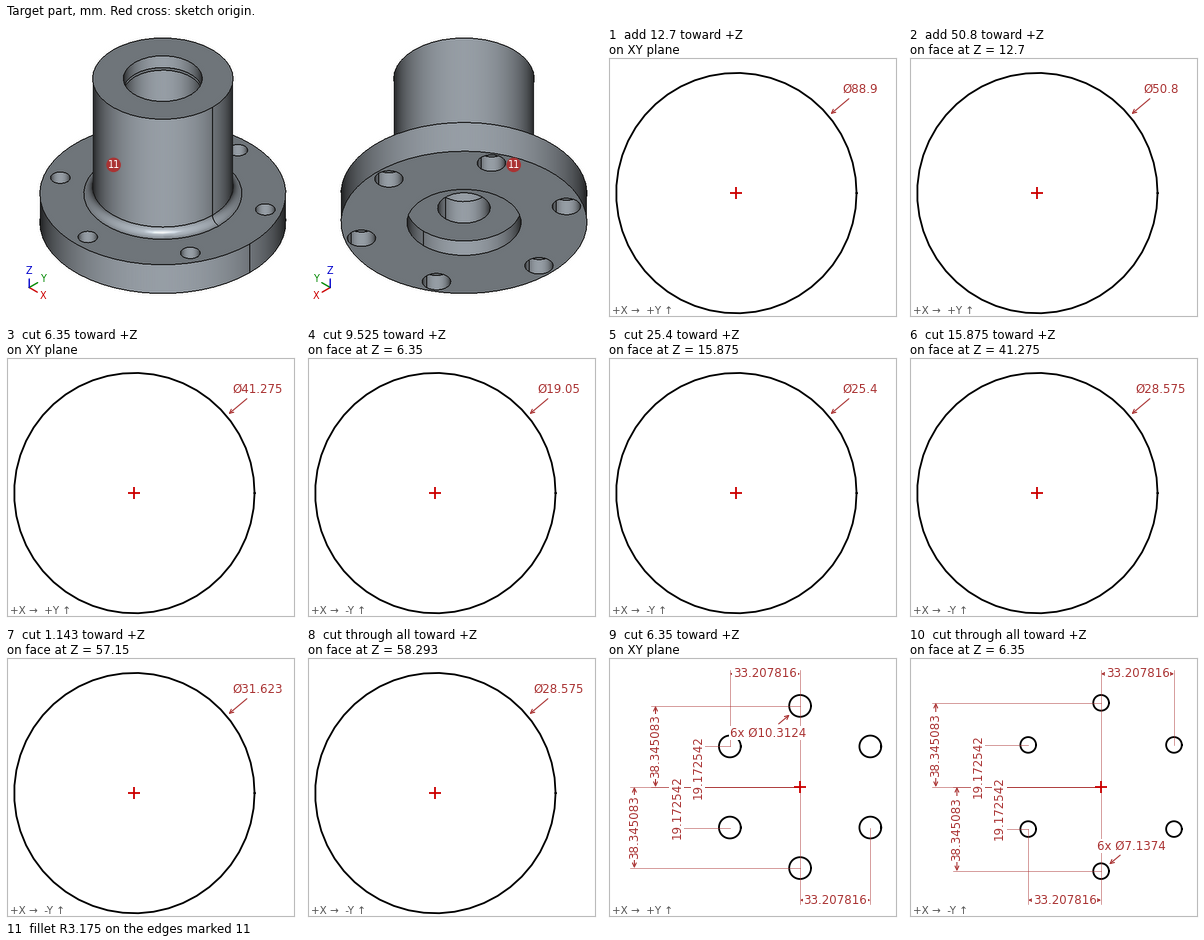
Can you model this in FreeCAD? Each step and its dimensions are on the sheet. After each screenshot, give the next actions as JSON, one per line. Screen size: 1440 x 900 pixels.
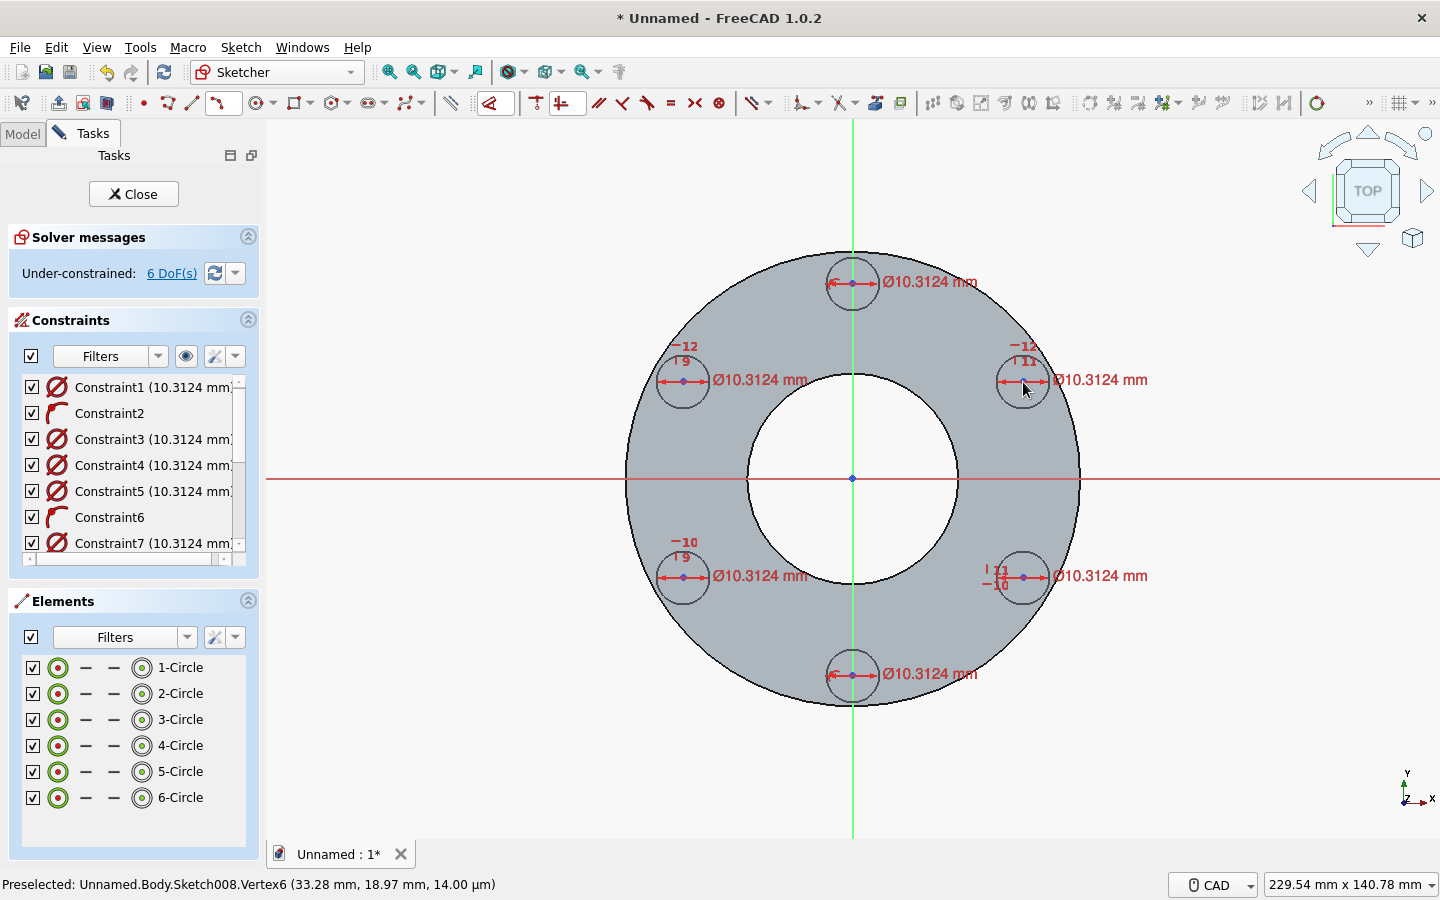
{"action": "key", "text": "d"}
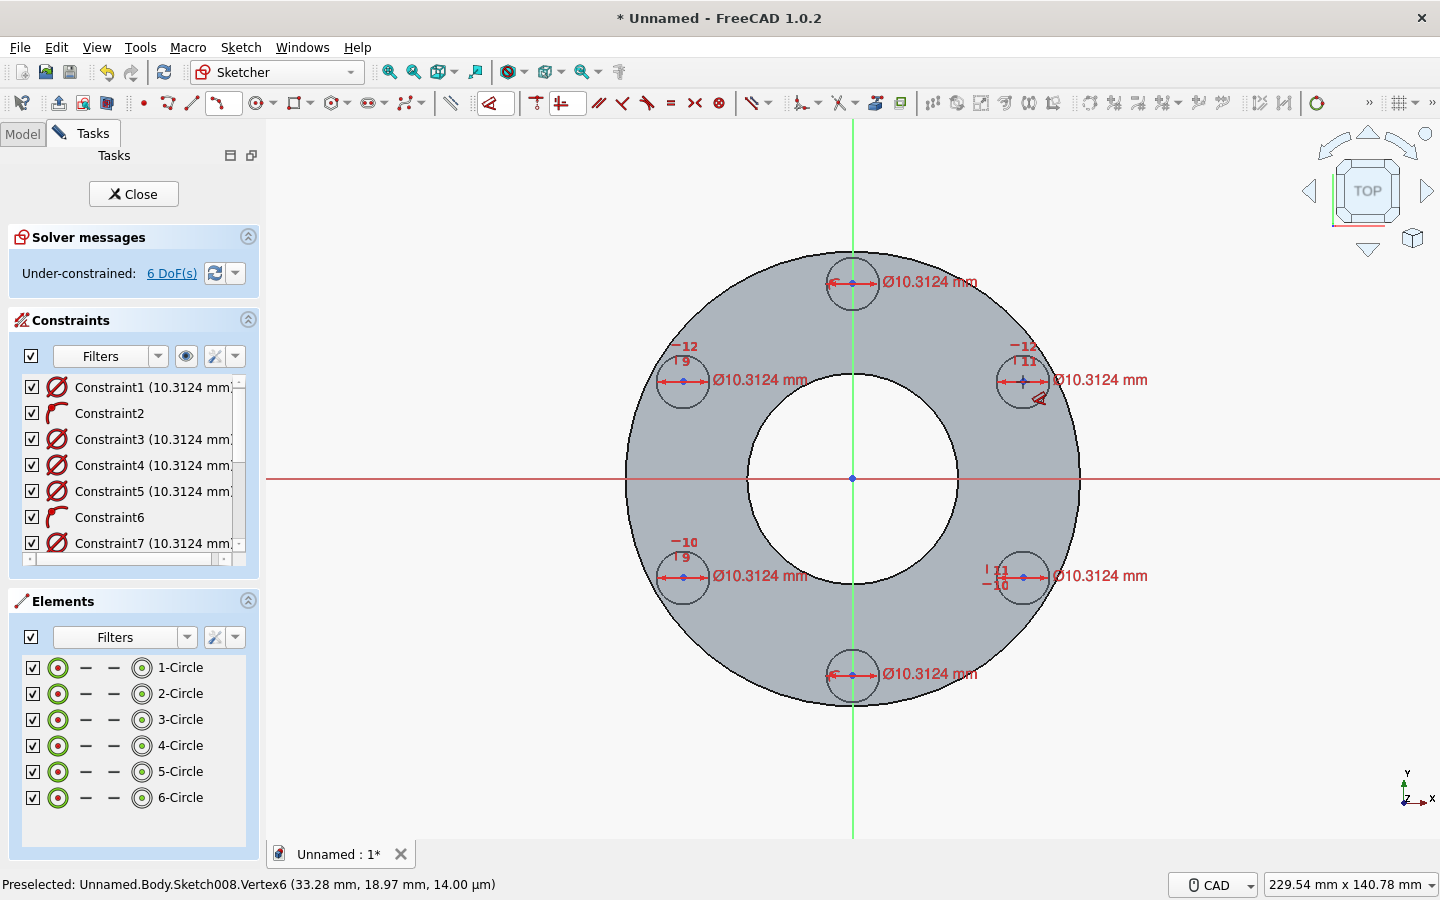
{"action": "left_click", "coordinate": [853, 284]}
{"action": "left_click", "coordinate": [887, 381]}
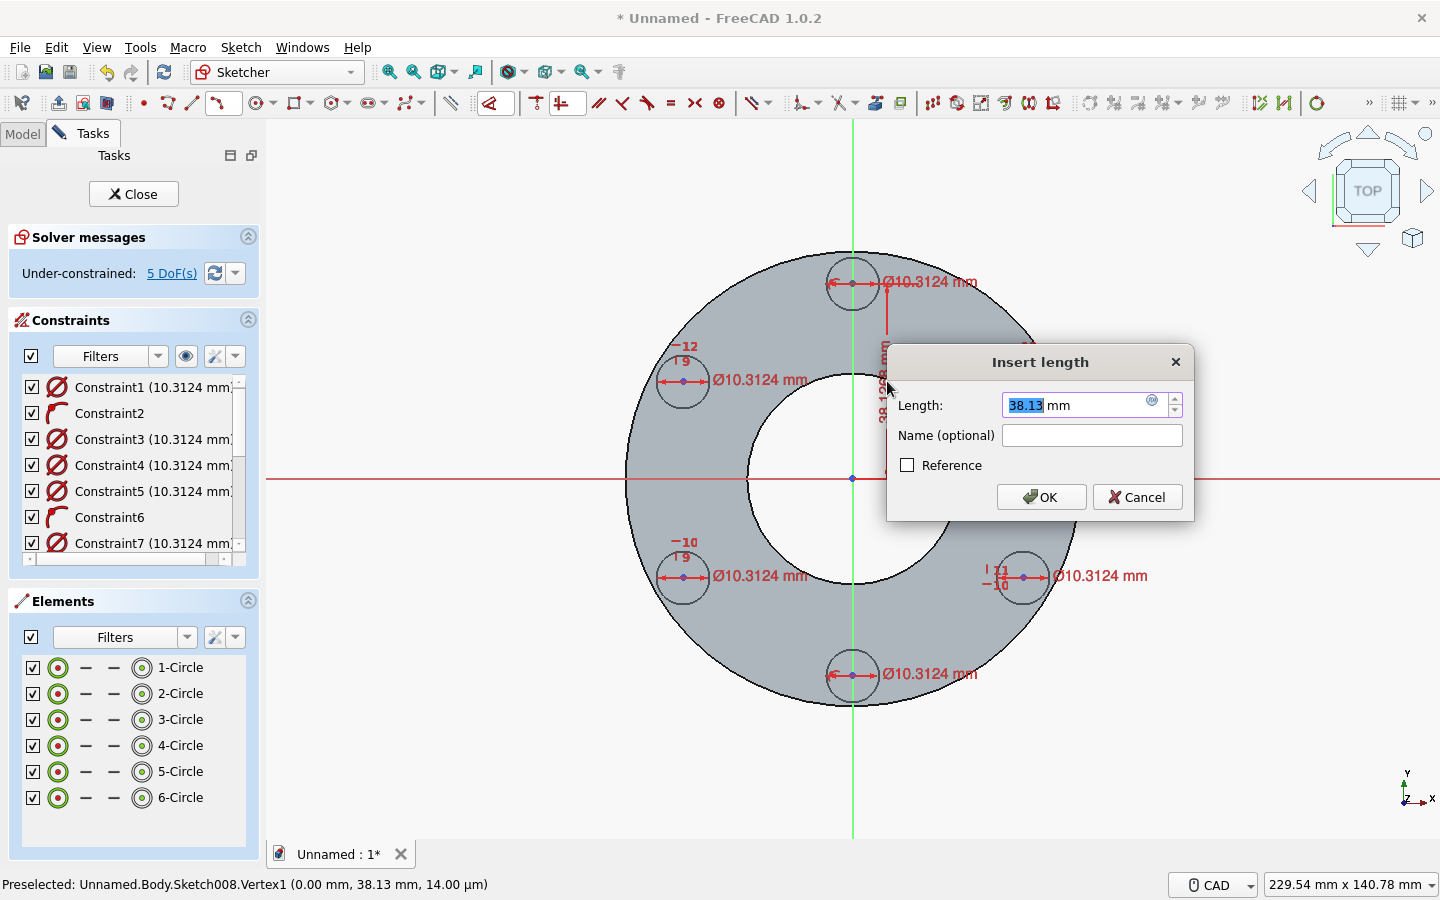
{"action": "type", "text": "38.345083"}
{"action": "key", "text": "Return"}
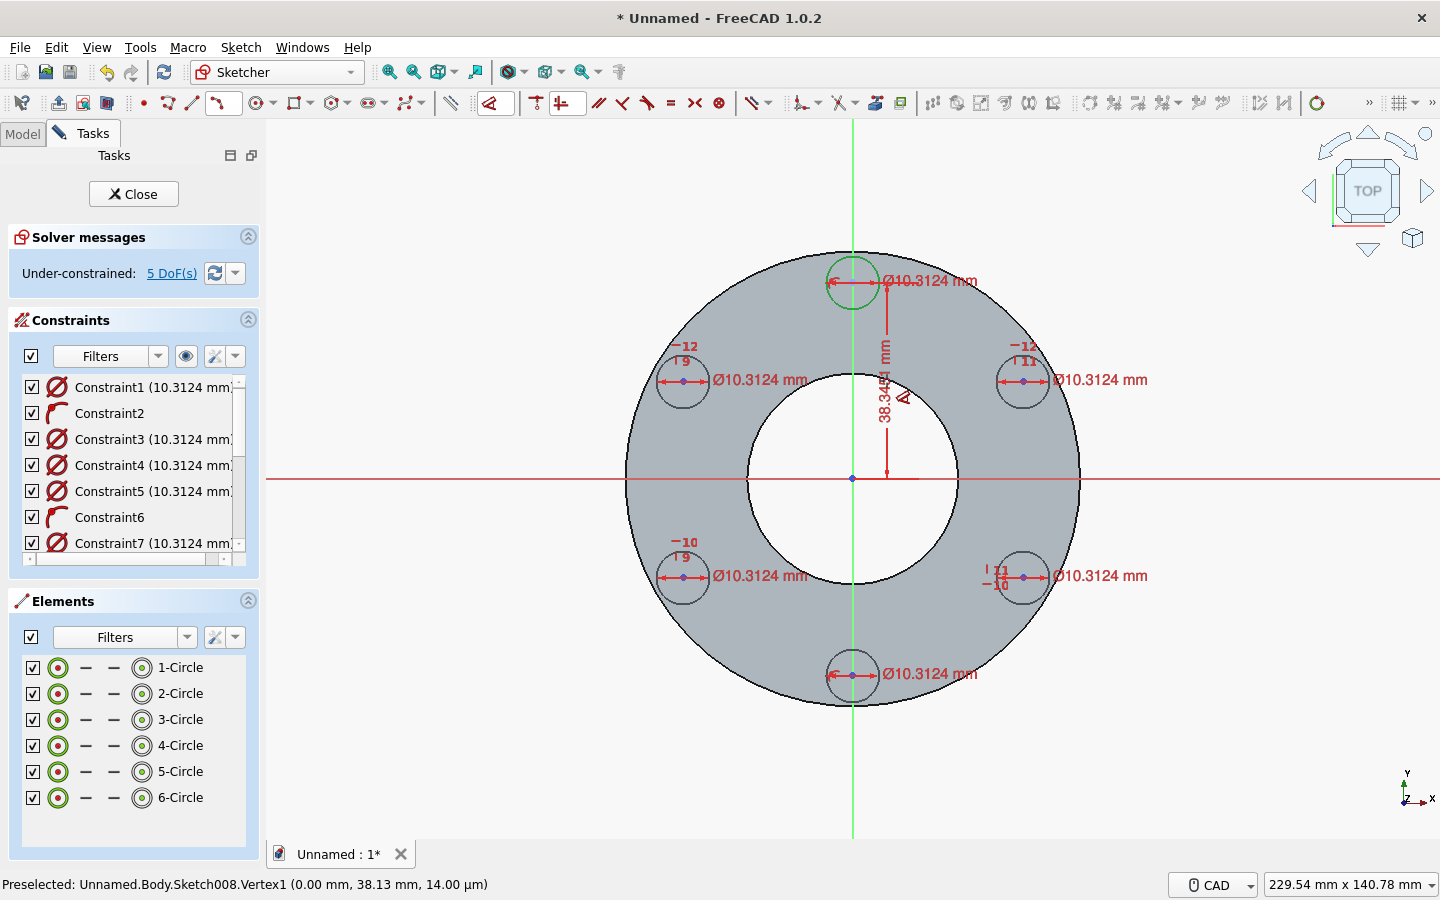
{"action": "left_click", "coordinate": [683, 382]}
{"action": "left_click", "coordinate": [768, 348]}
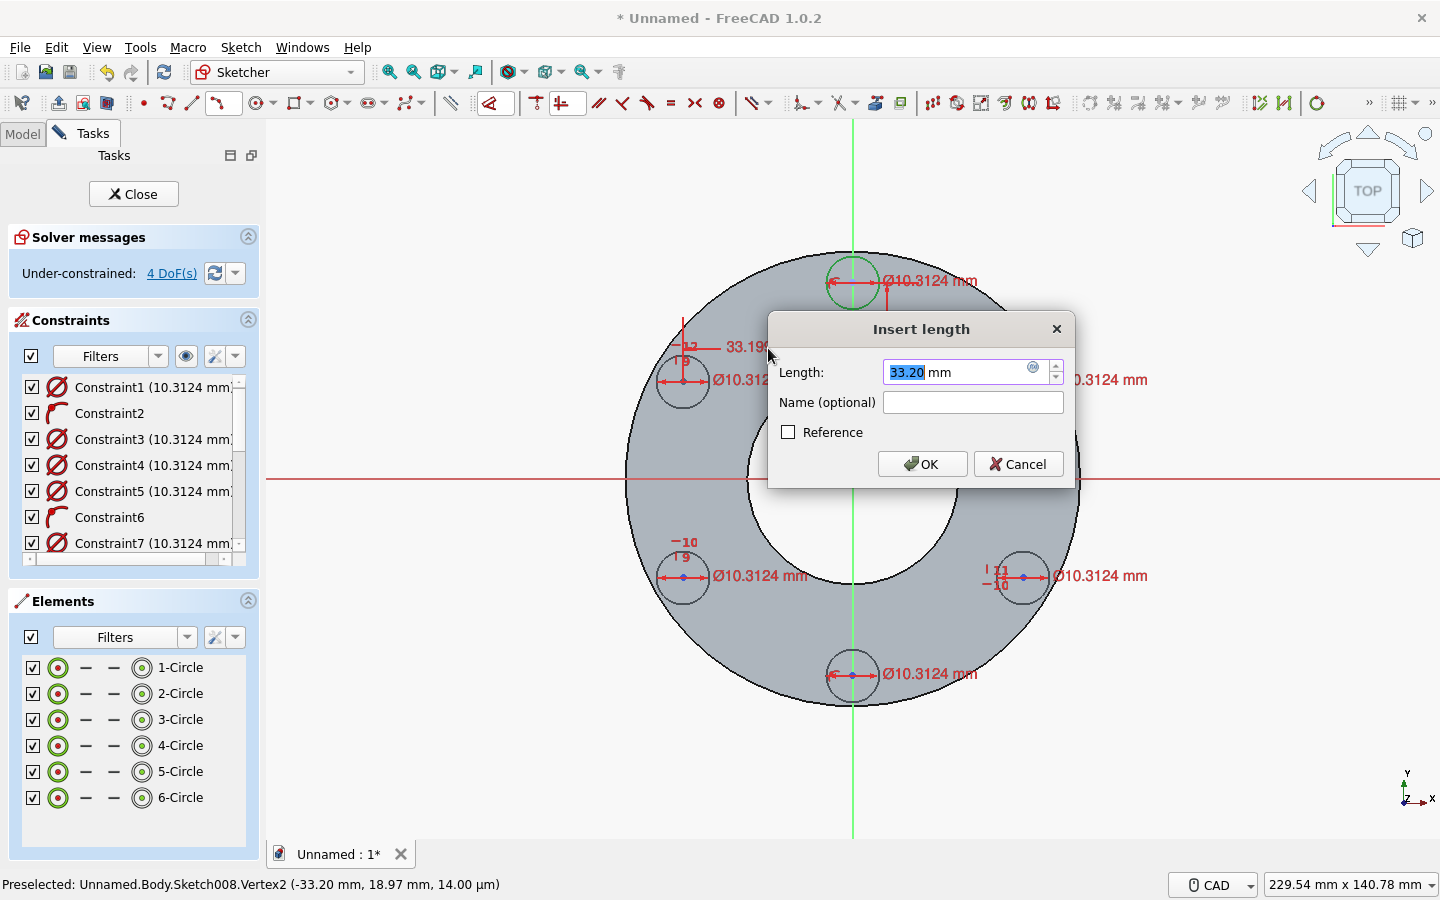
{"action": "type", "text": "33.207816"}
{"action": "key", "text": "Return"}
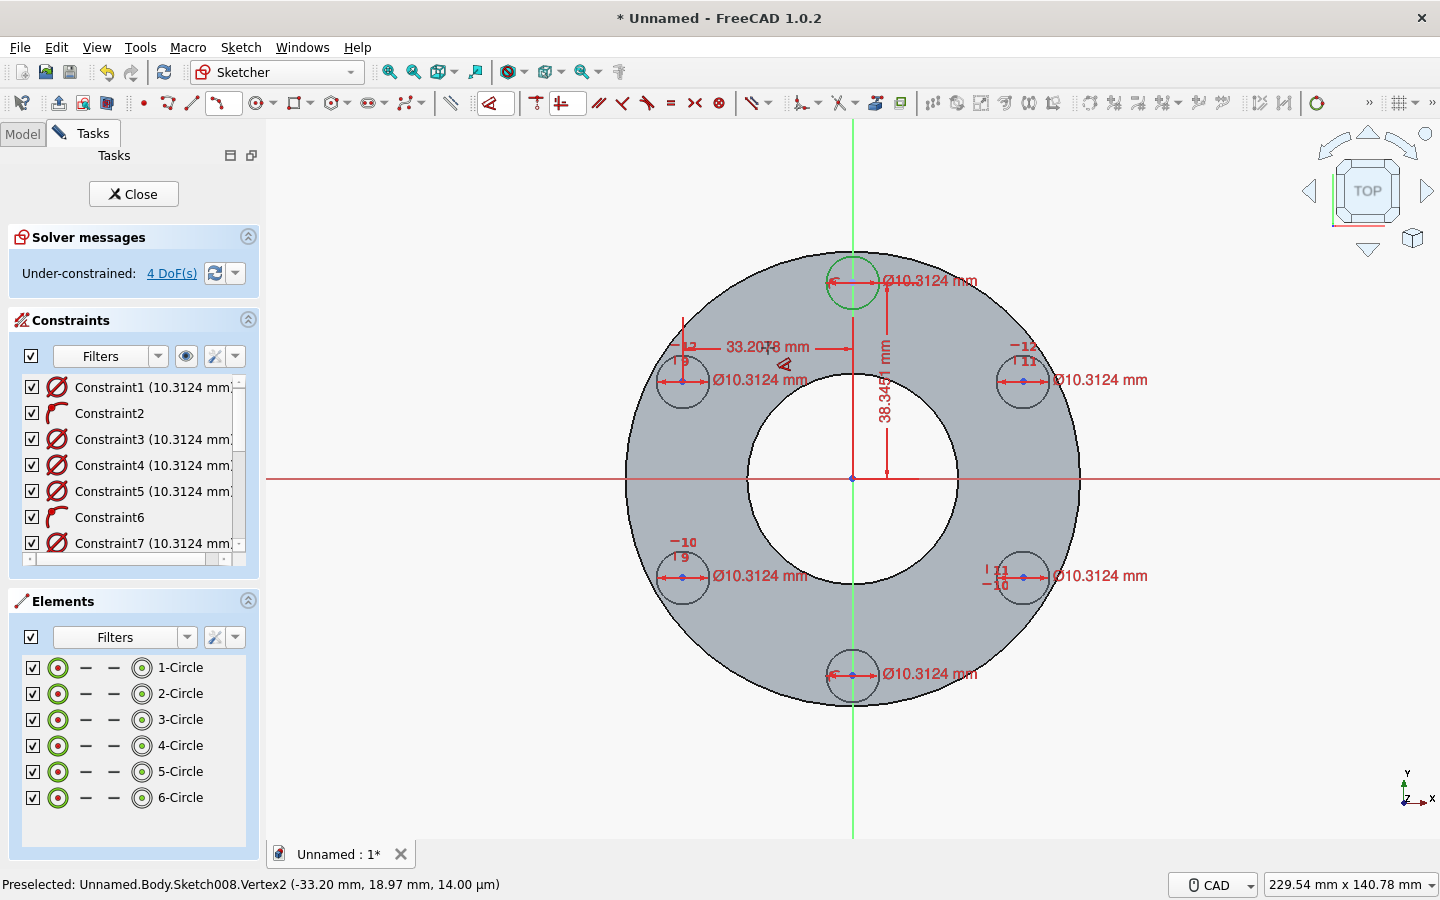
{"action": "left_click", "coordinate": [683, 382]}
{"action": "left_click", "coordinate": [649, 430]}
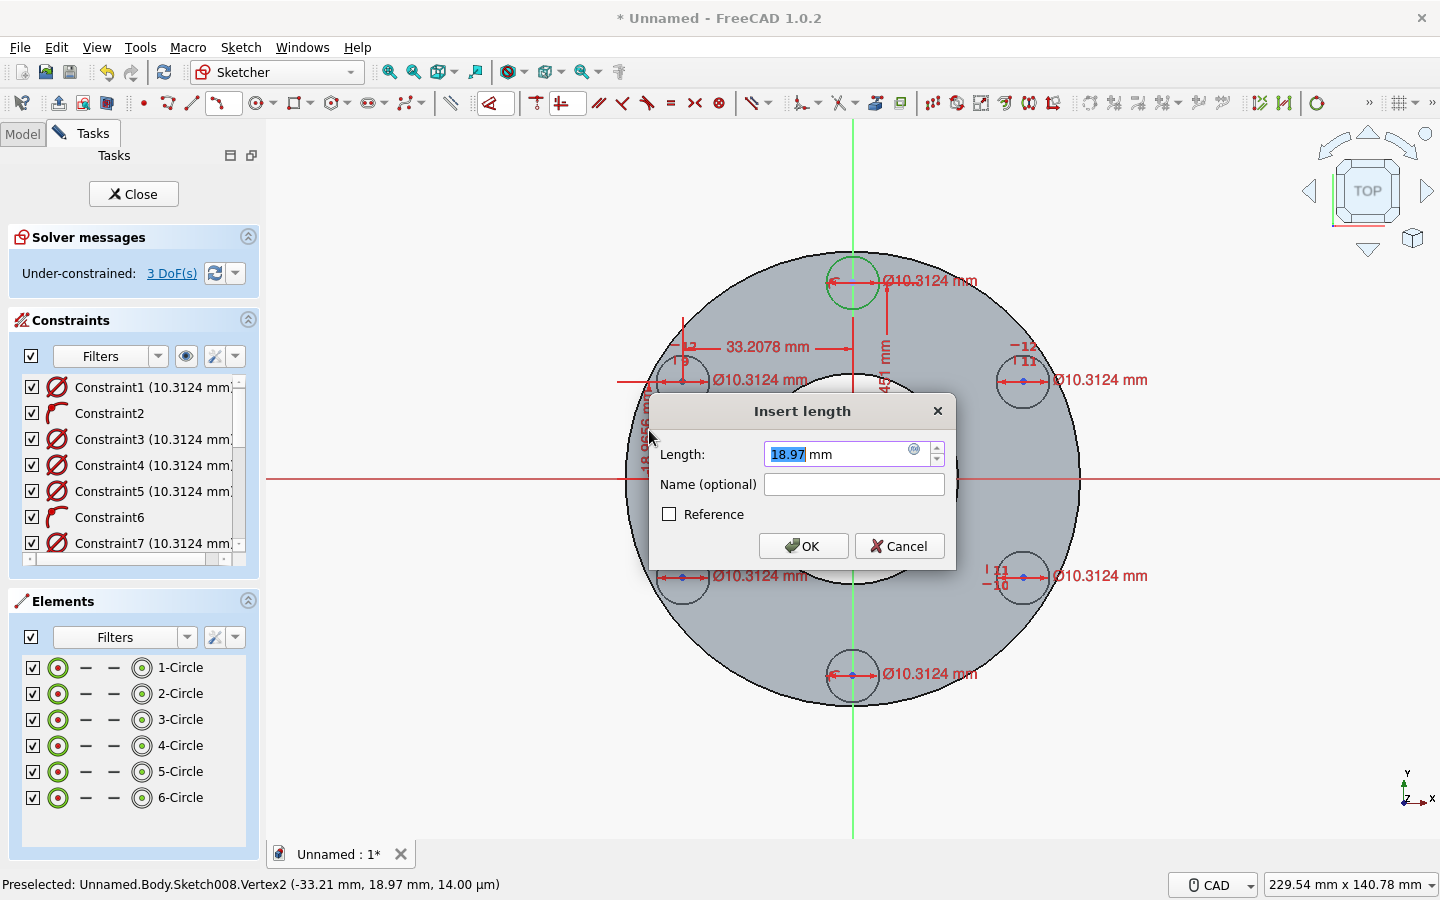
{"action": "type", "text": "19.172542"}
{"action": "key", "text": "Return"}